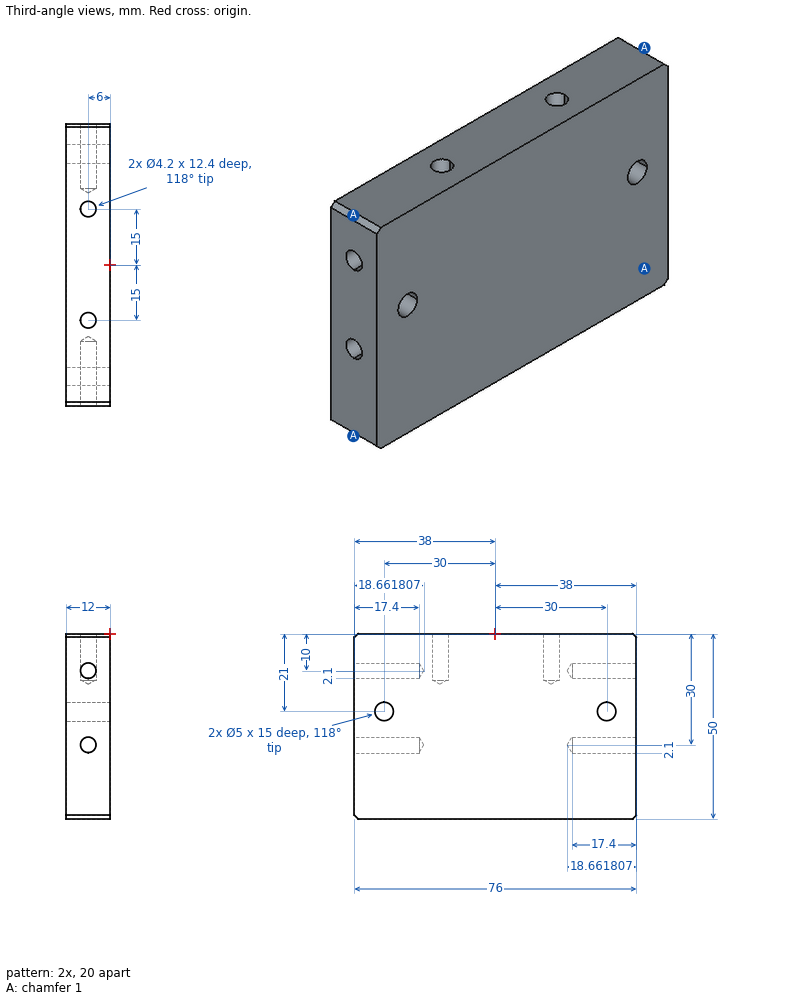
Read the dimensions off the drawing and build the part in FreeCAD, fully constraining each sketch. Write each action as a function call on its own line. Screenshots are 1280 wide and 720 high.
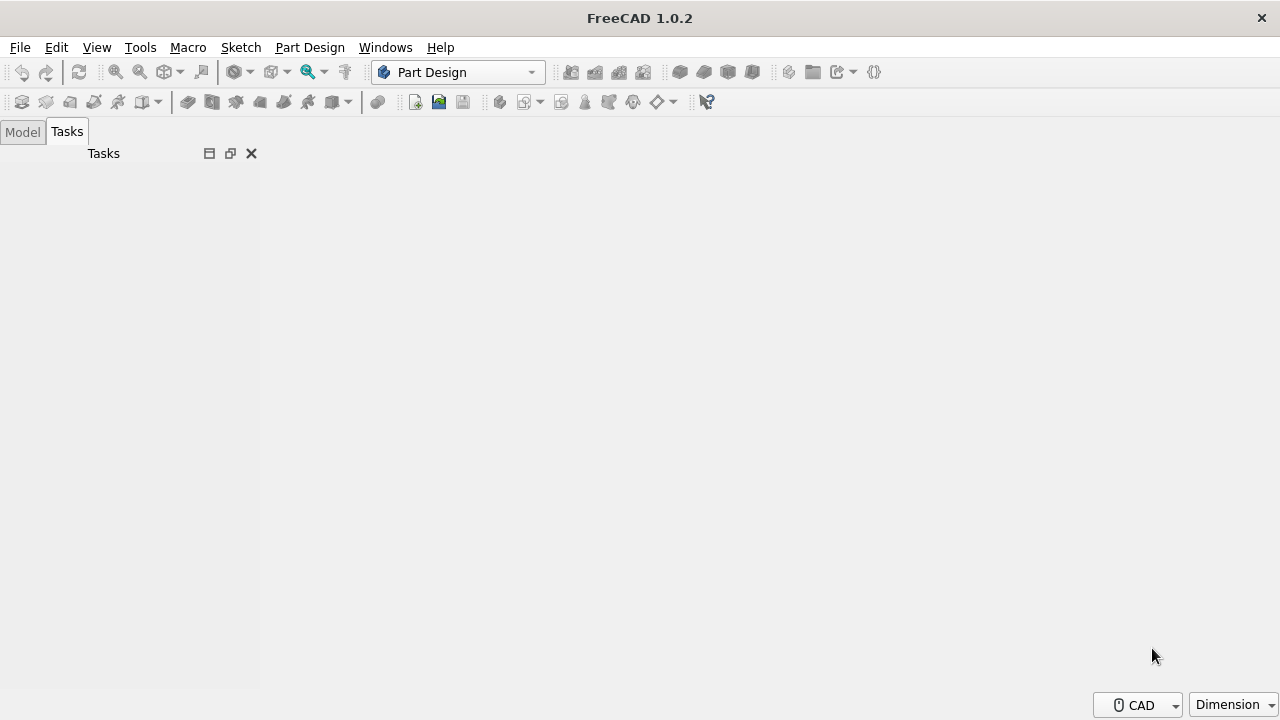
click(416, 102)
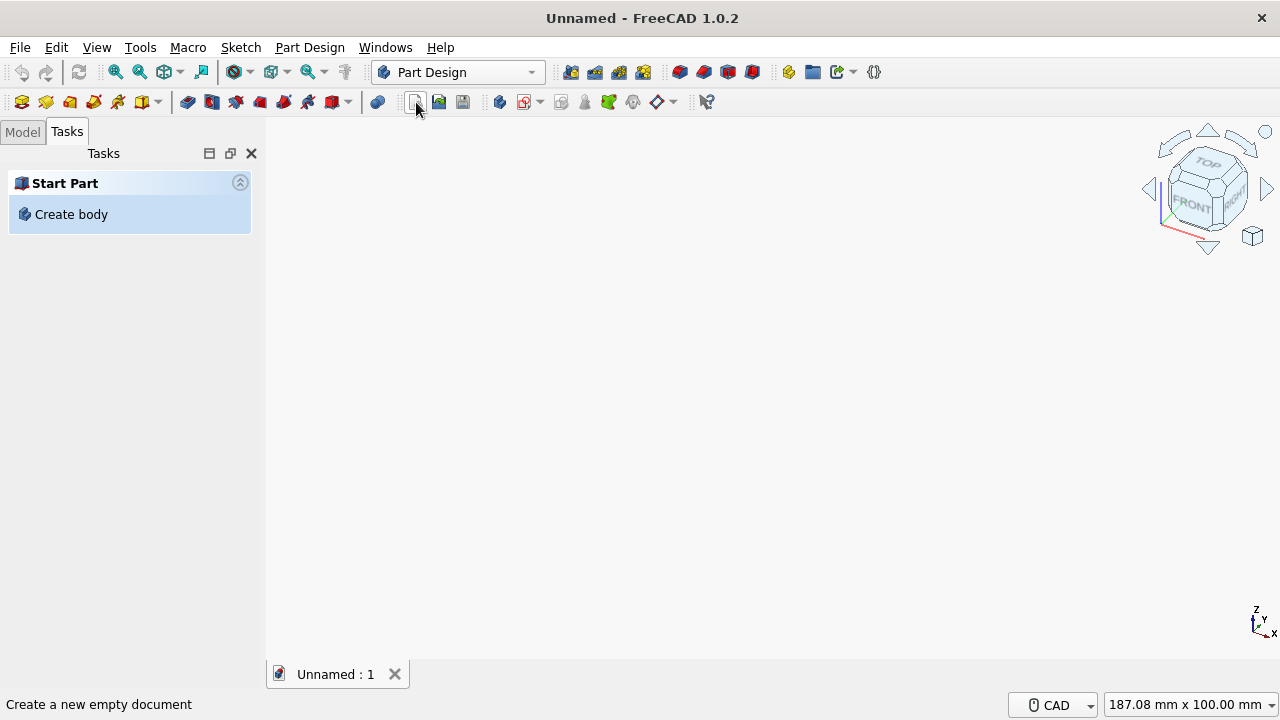
click(524, 102)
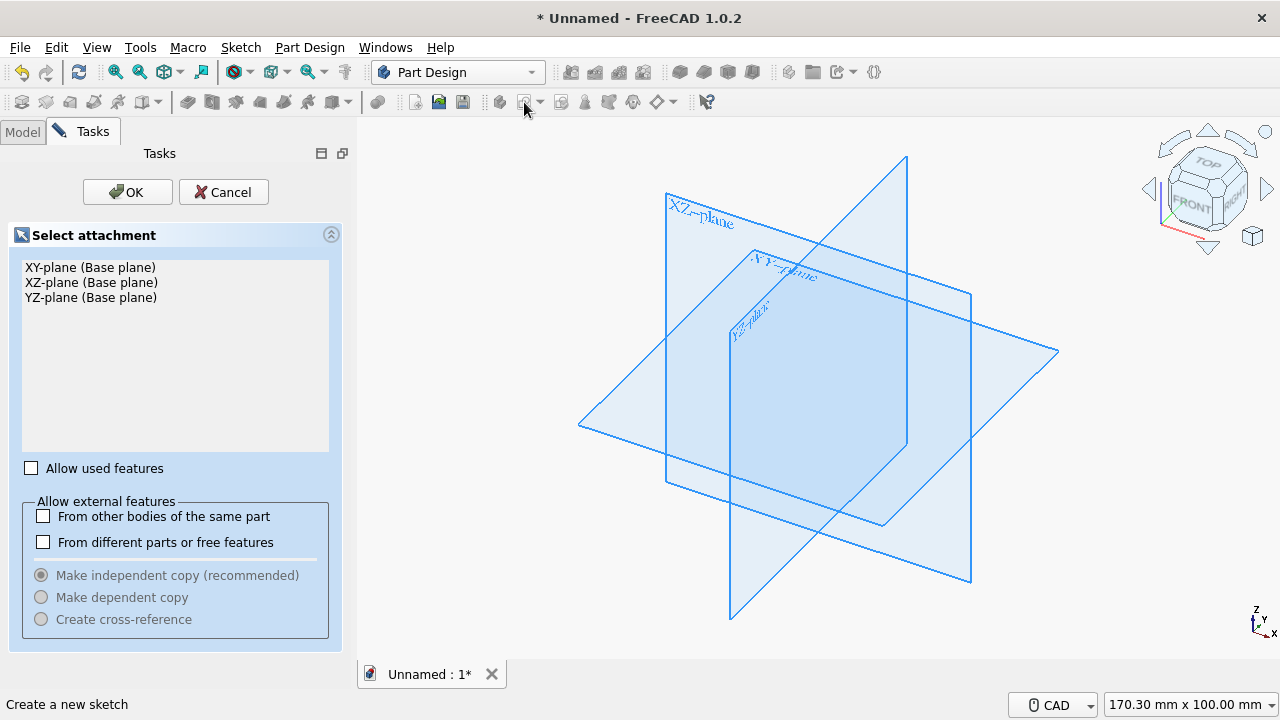
click(82, 298)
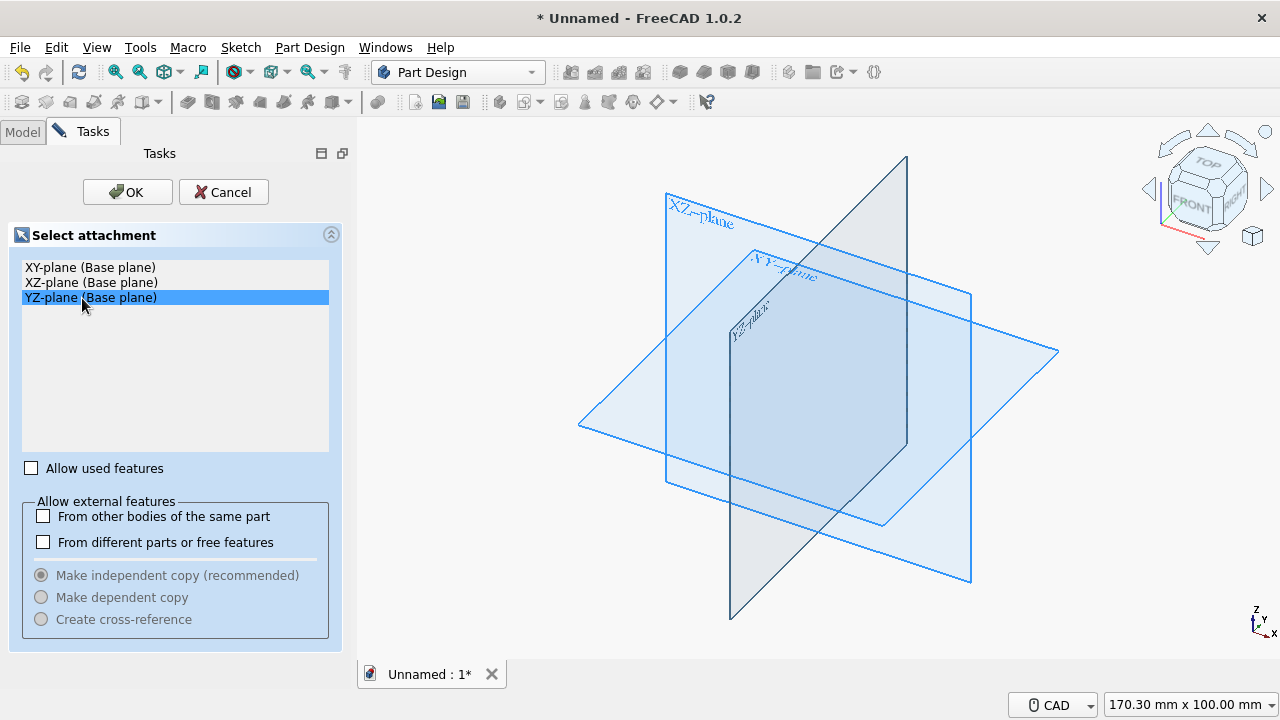
click(128, 192)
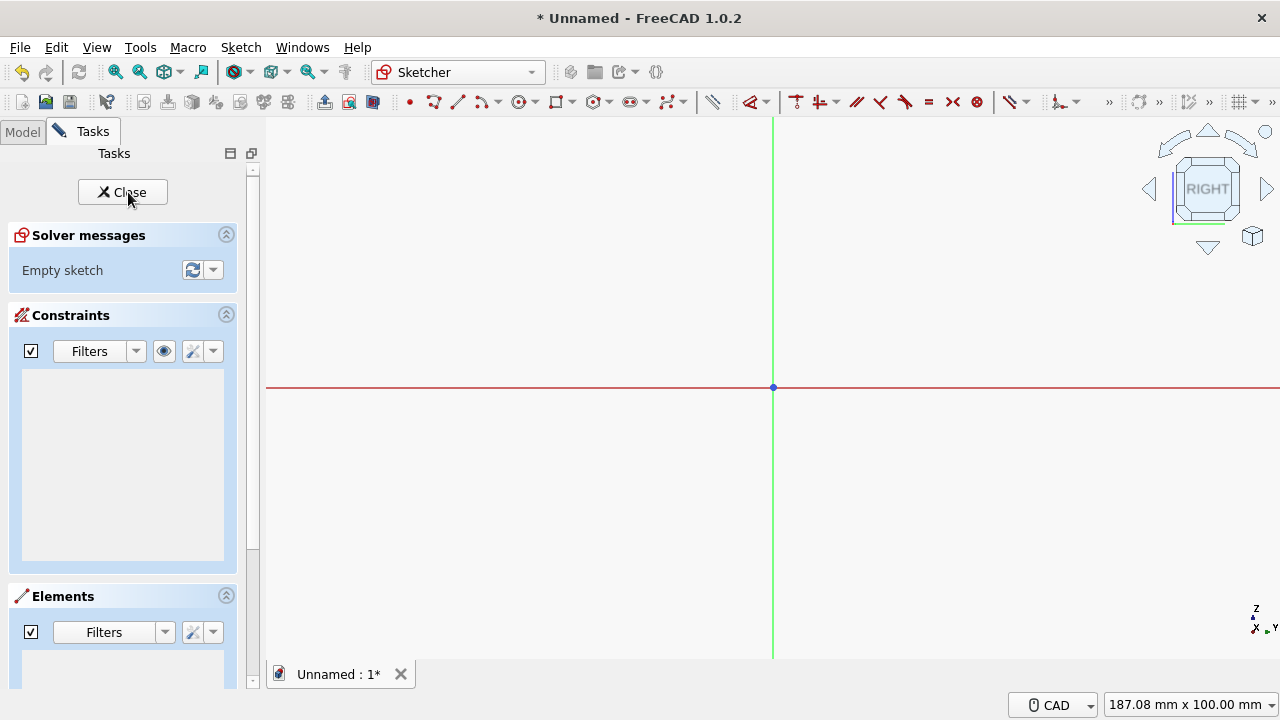
scroll(395, 145, down, 1)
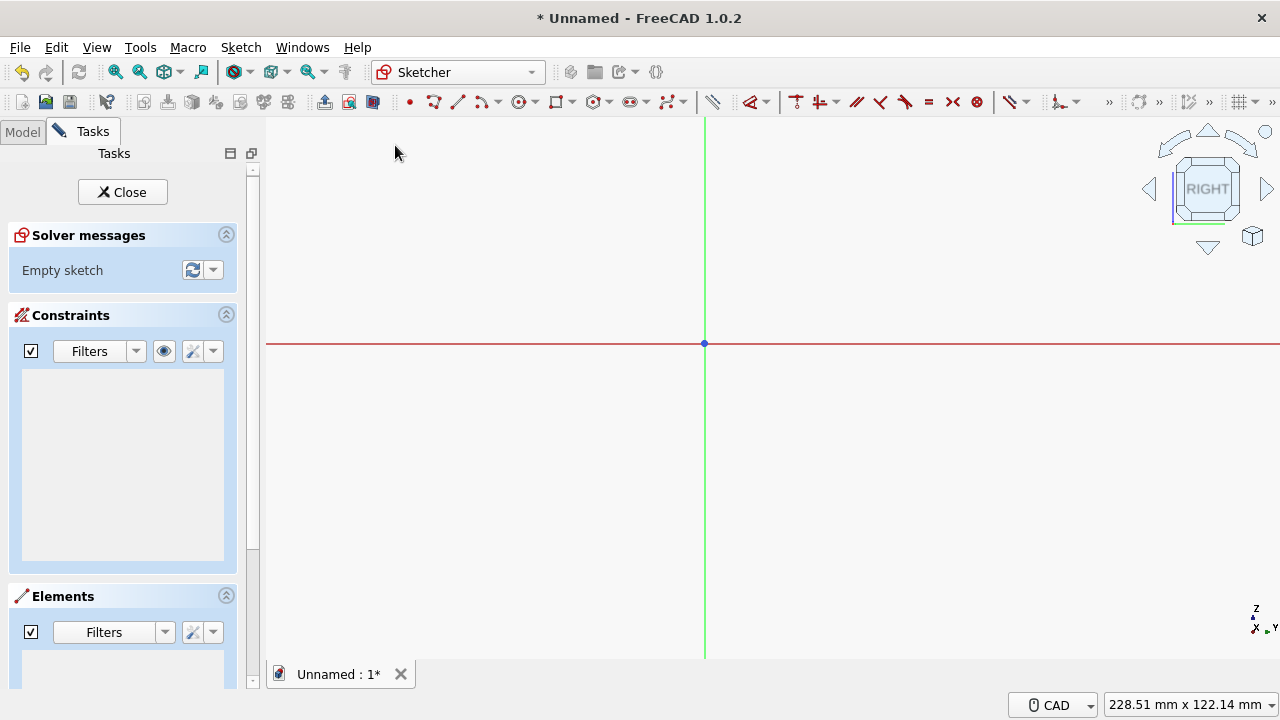
scroll(705, 591, up, 2)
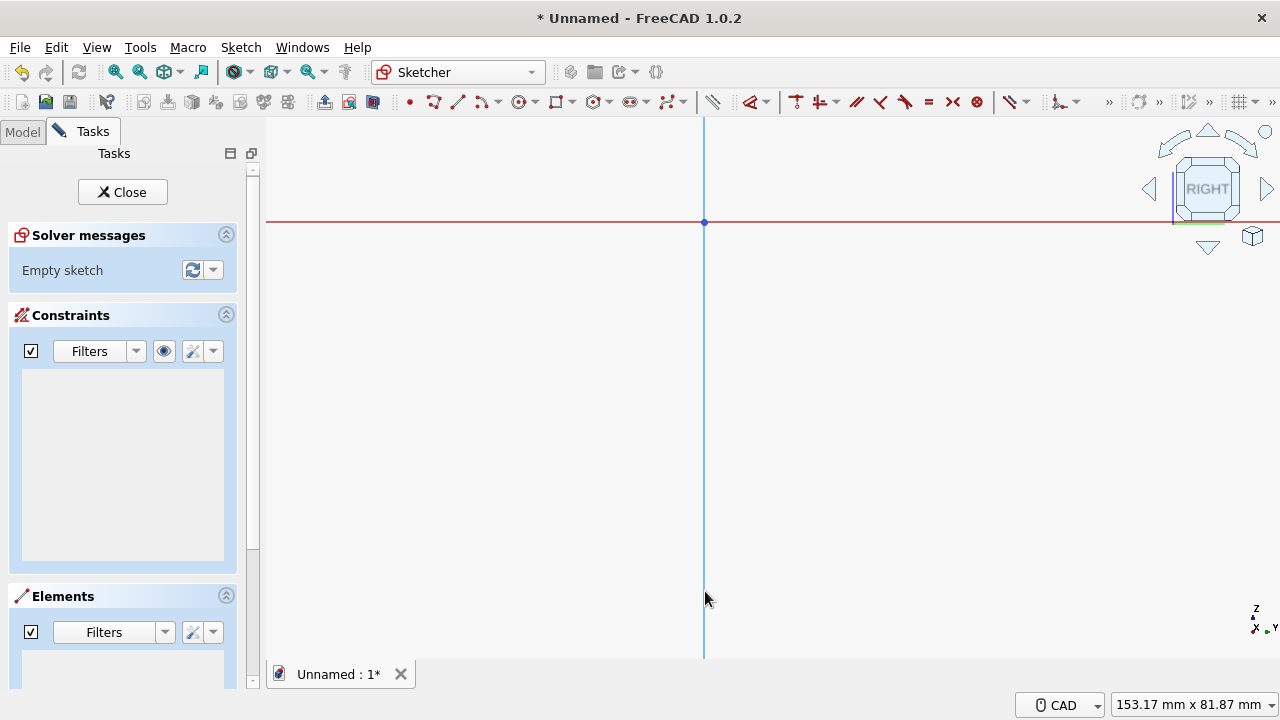
click(556, 102)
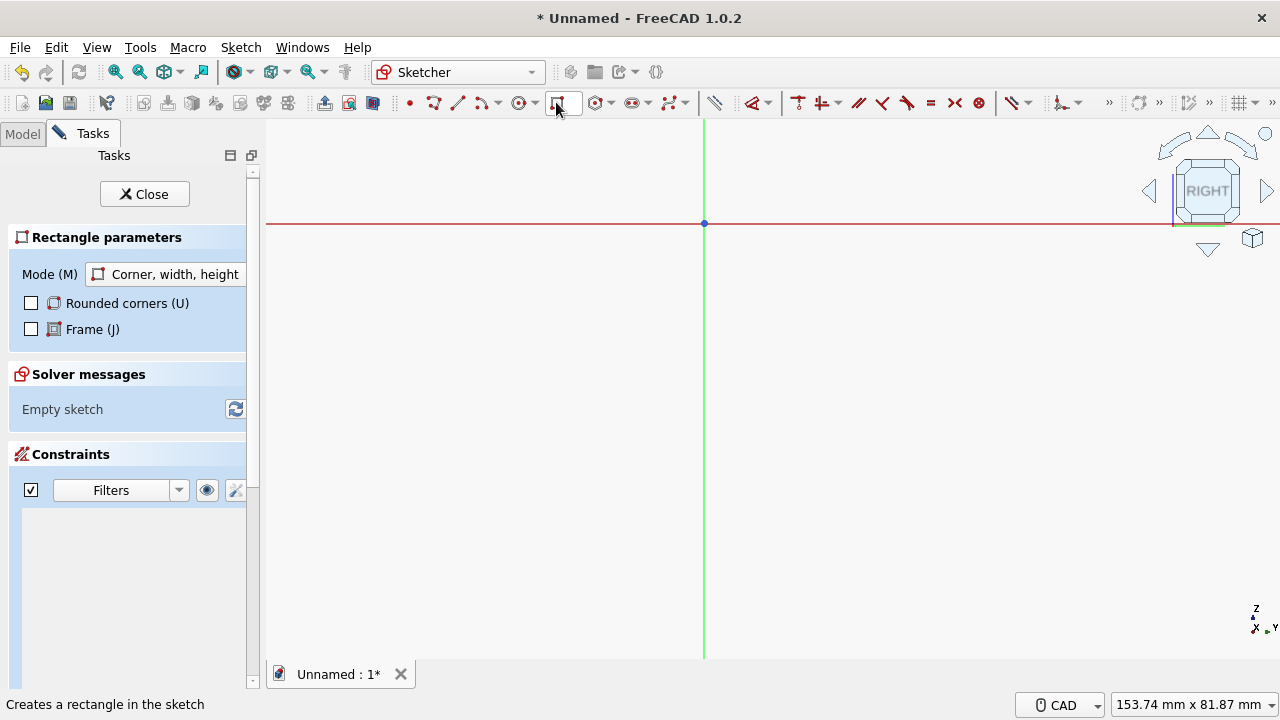
click(454, 224)
move(955, 553)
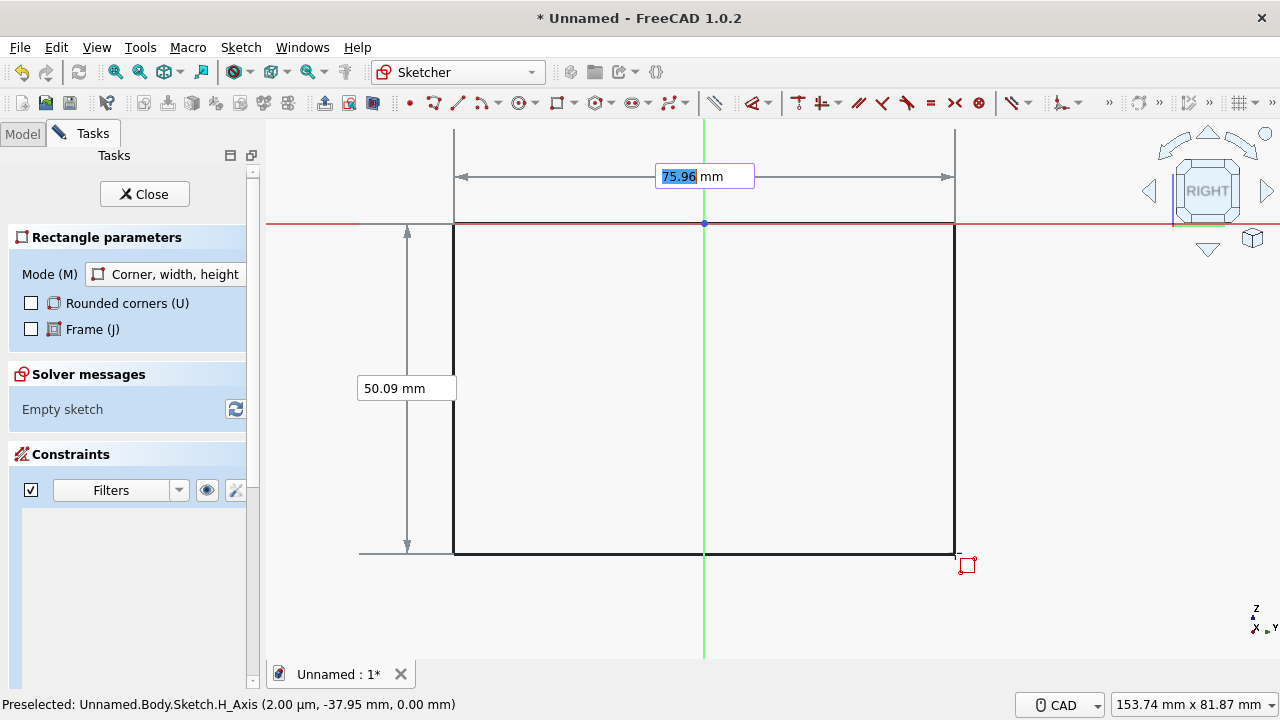
text(76)
key(Tab)
text(50)
key(Return)
key(Escape)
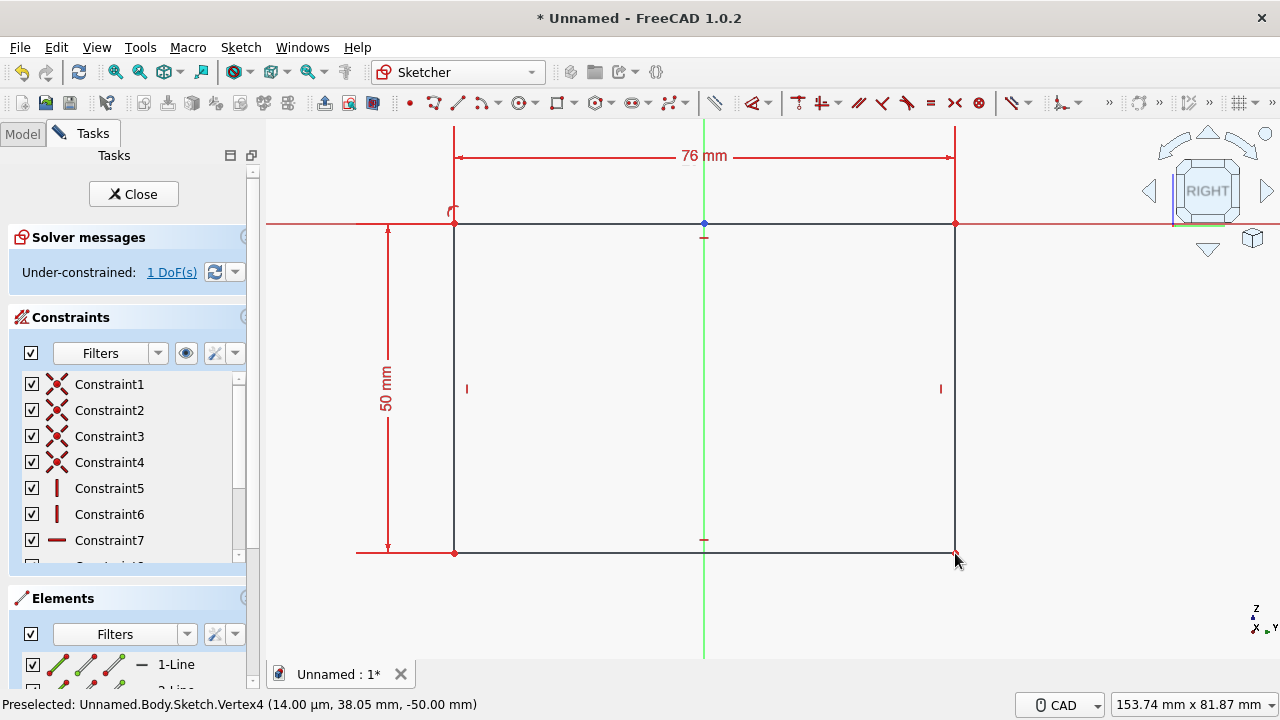
click(454, 224)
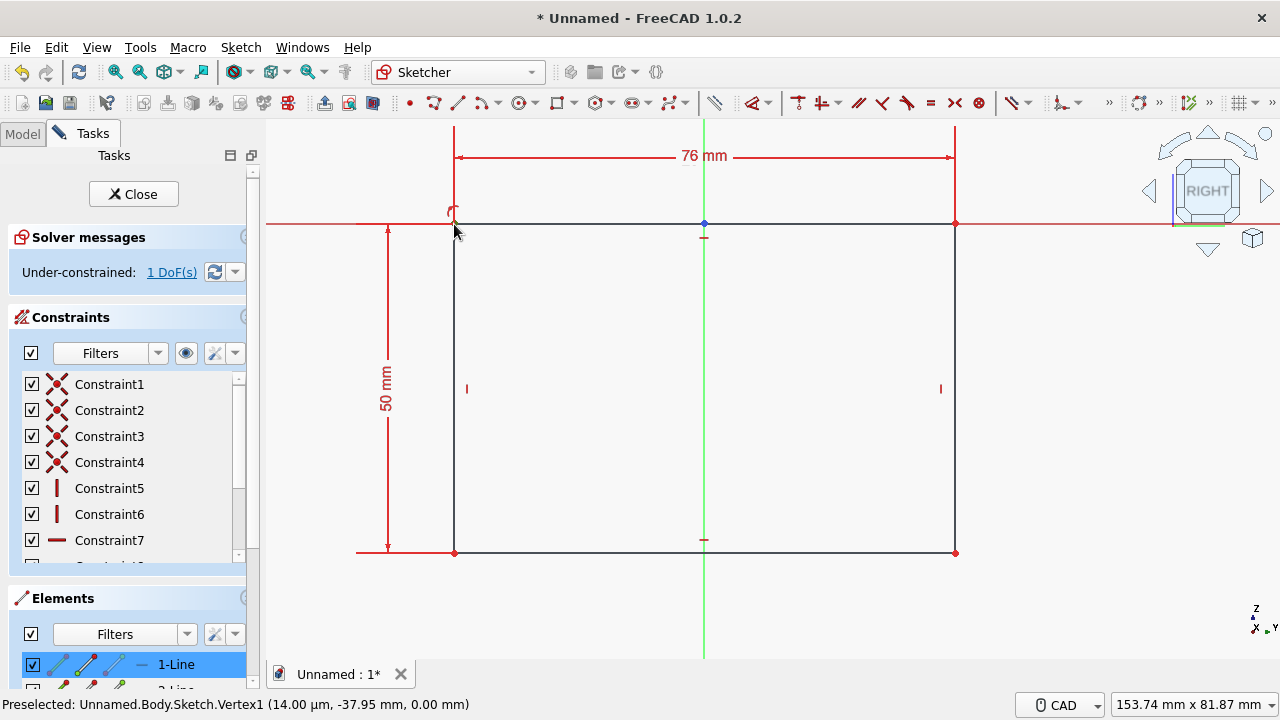
click(770, 104)